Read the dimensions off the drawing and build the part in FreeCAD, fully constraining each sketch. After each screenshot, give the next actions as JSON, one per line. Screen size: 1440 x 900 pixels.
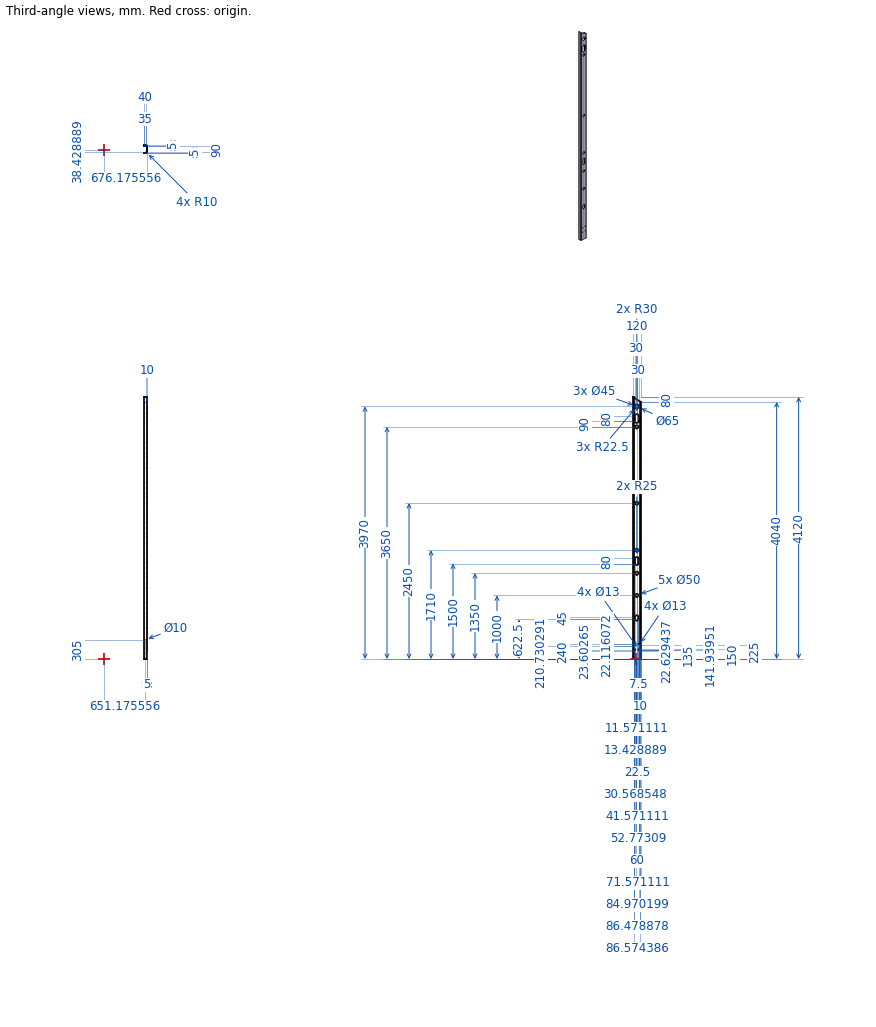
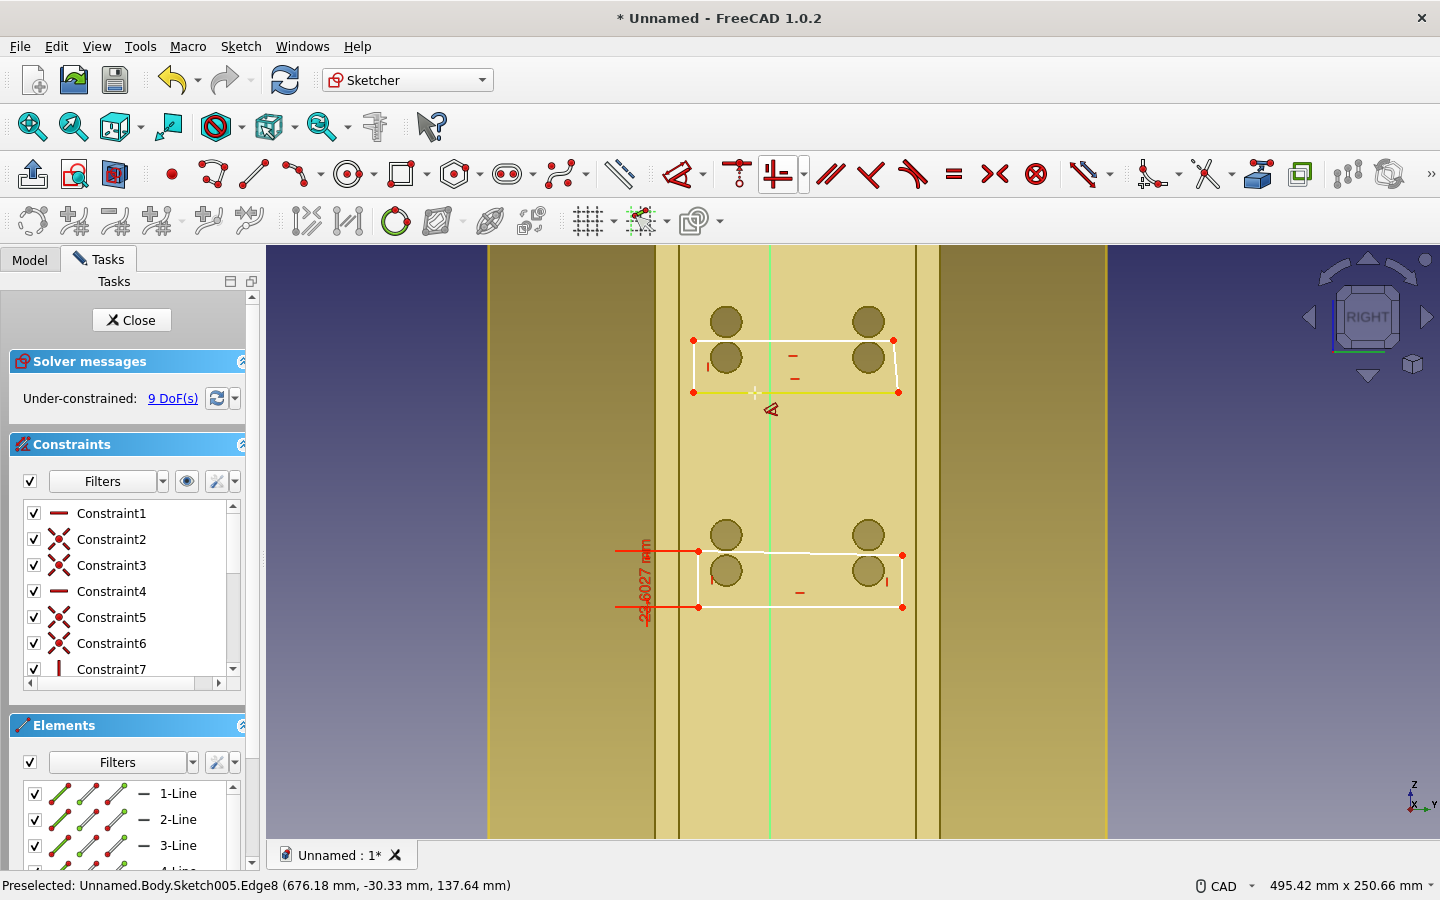
{"action": "left_click", "coordinate": [755, 393]}
{"action": "left_click", "coordinate": [796, 359]}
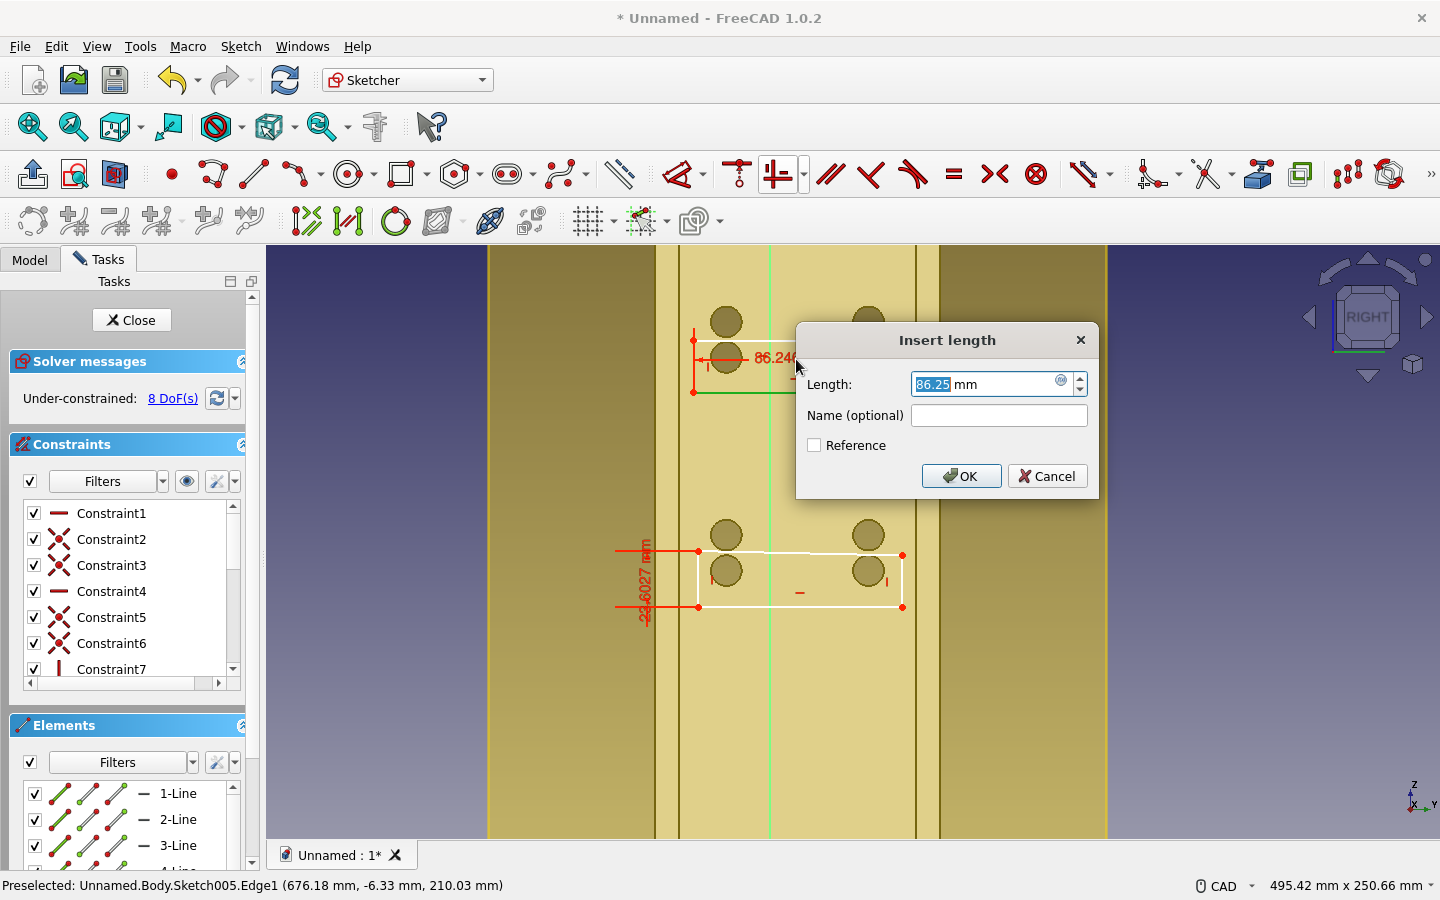
{"action": "type", "text": "86.478878"}
{"action": "key", "text": "Return"}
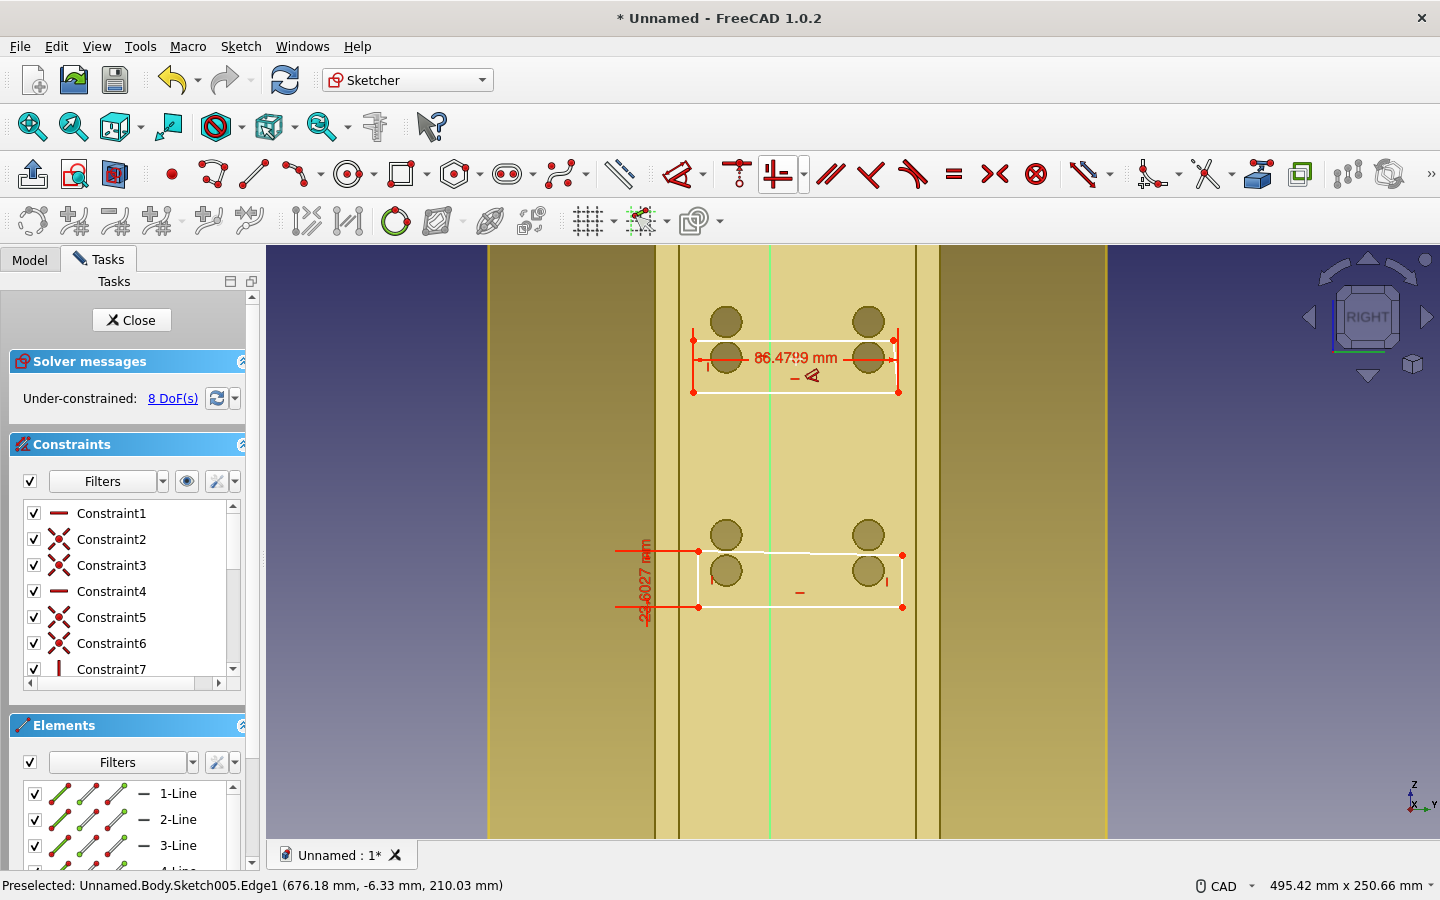
{"action": "left_click", "coordinate": [833, 341]}
{"action": "left_click", "coordinate": [793, 307]}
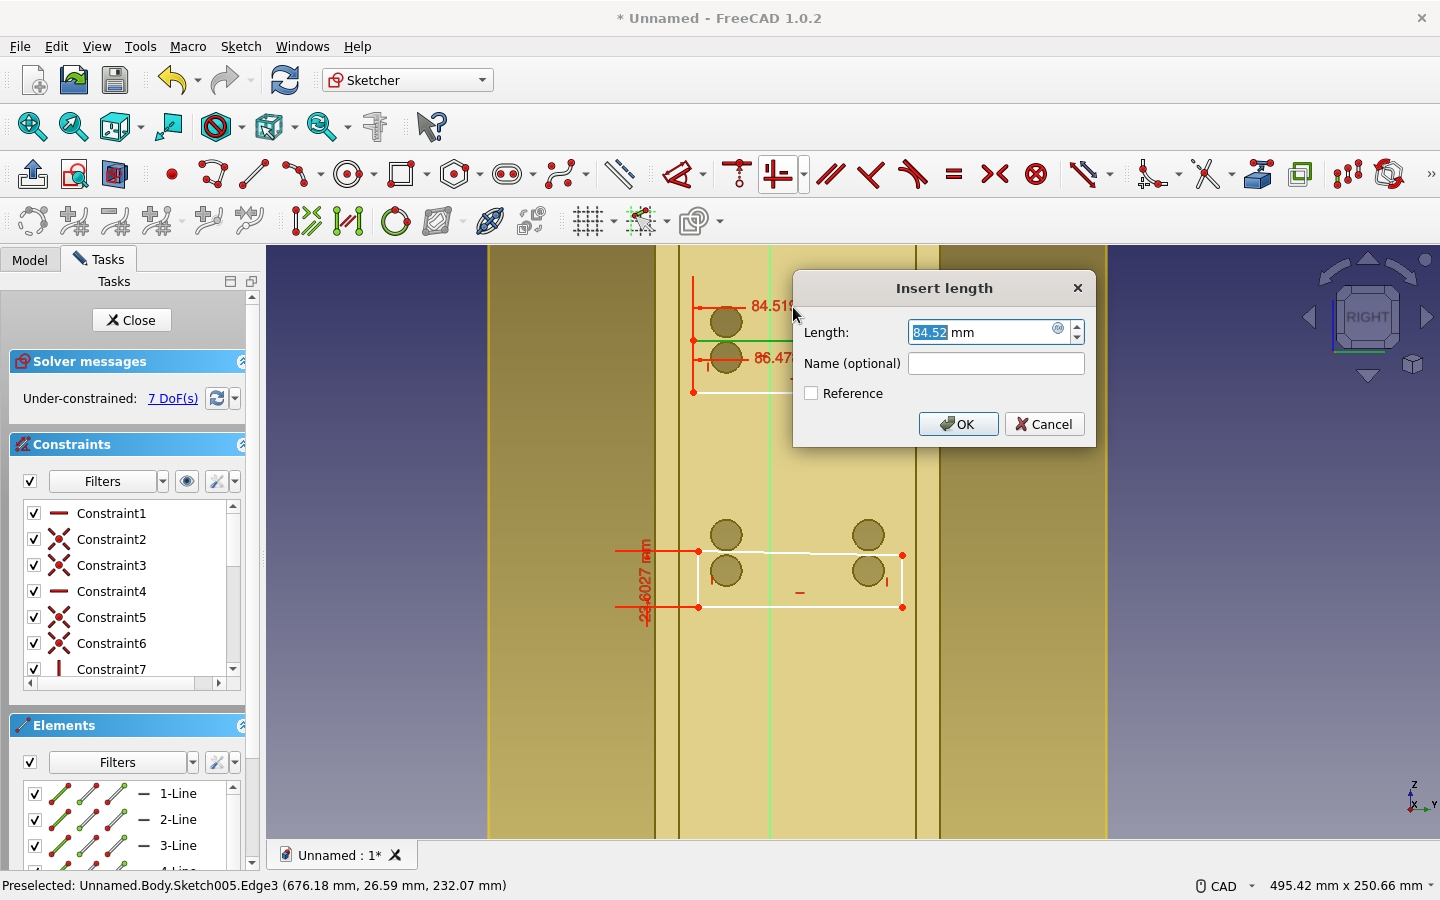
{"action": "type", "text": "84.970199"}
{"action": "key", "text": "Return"}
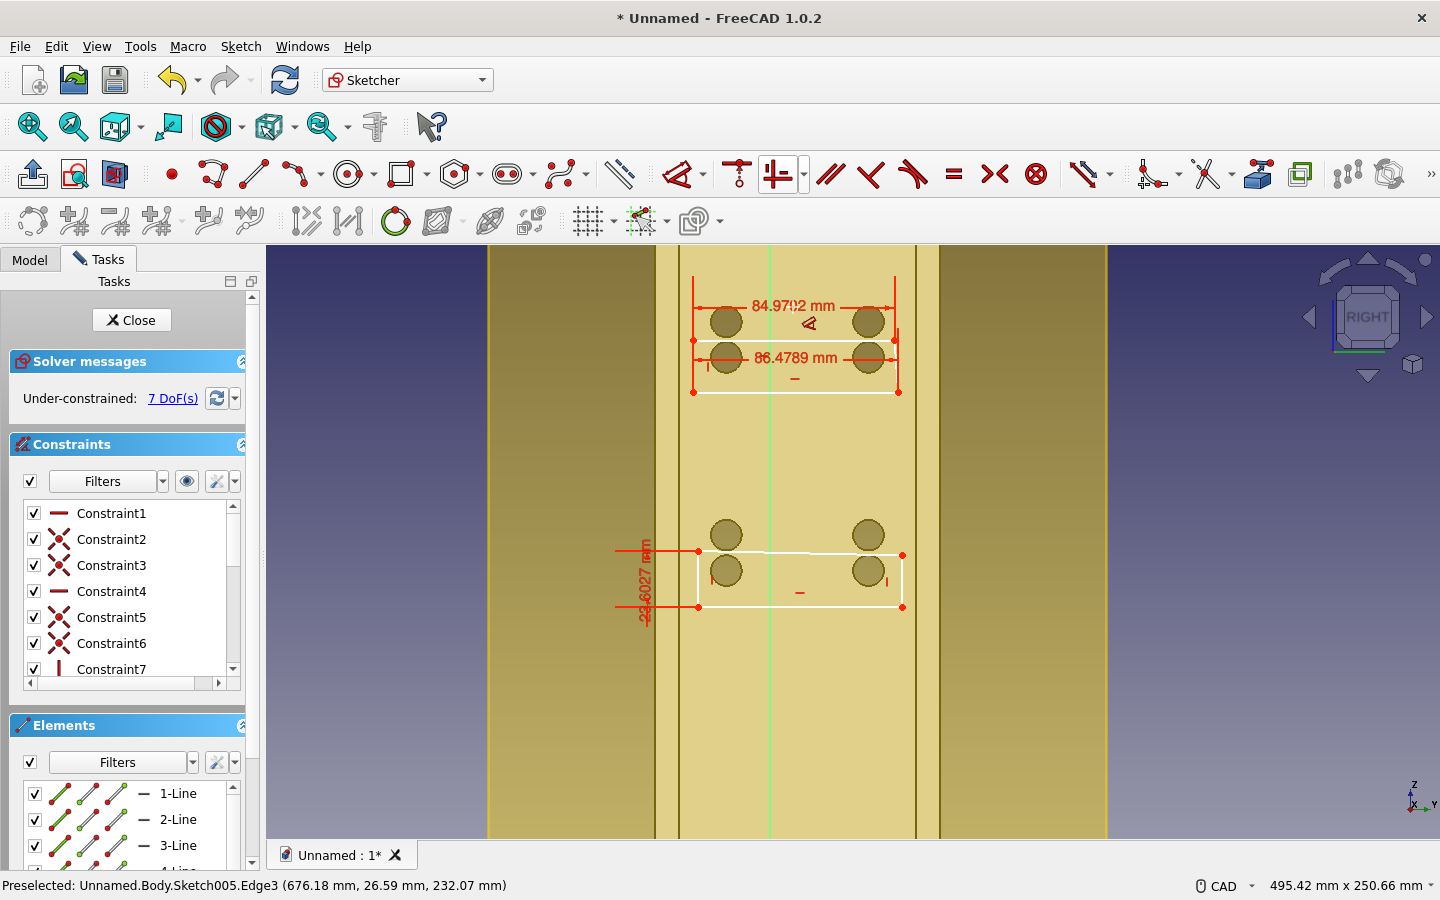
{"action": "left_click", "coordinate": [693, 356]}
{"action": "left_click", "coordinate": [659, 367]}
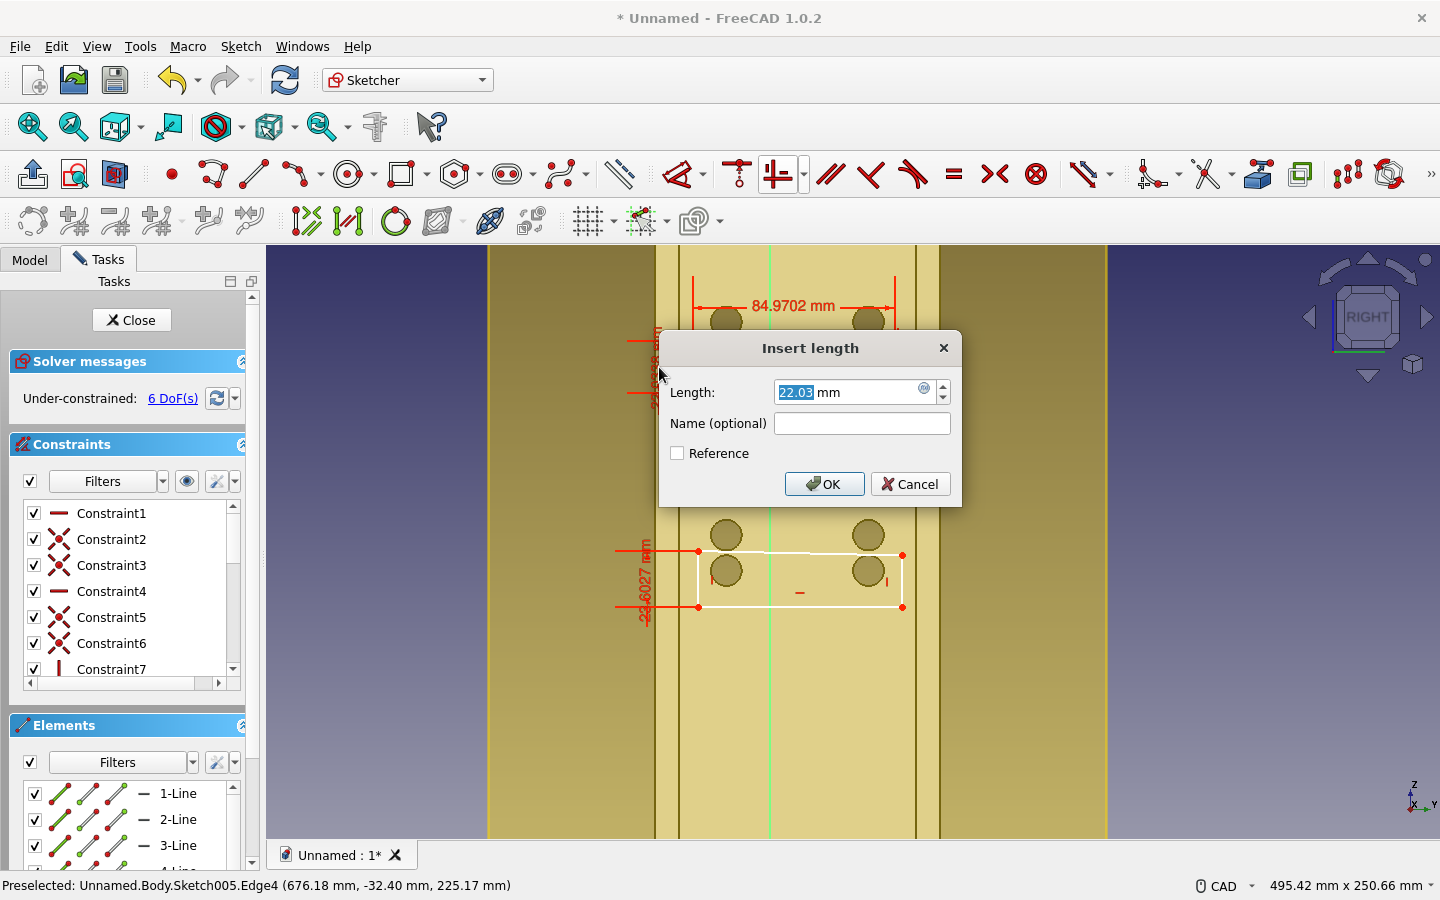
{"action": "type", "text": "22.116072"}
{"action": "key", "text": "Return"}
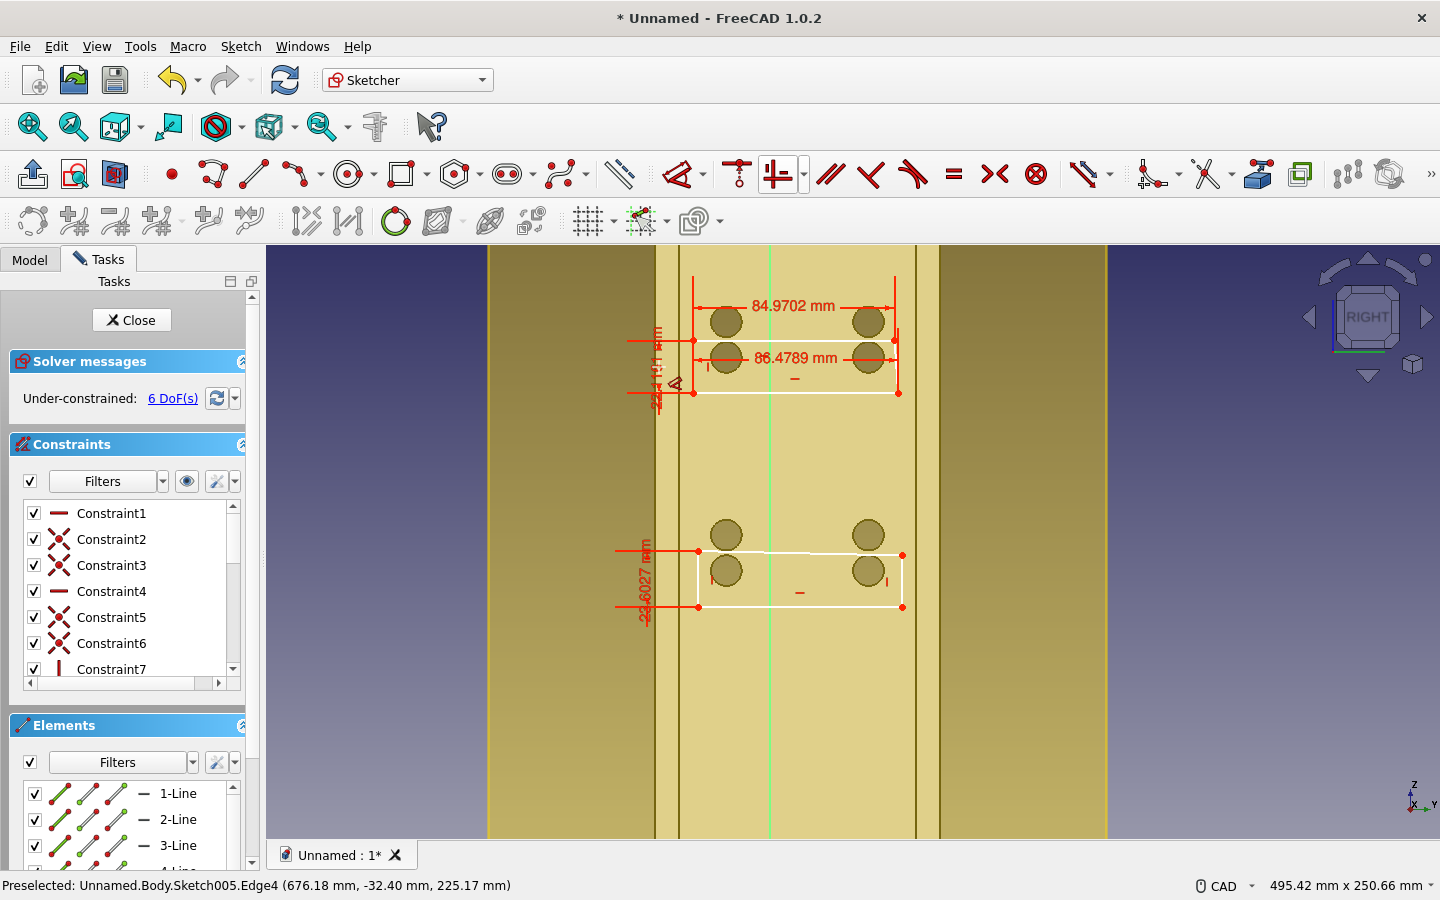
{"action": "scroll", "coordinate": [759, 607], "scroll_direction": "up", "scroll_amount": 2}